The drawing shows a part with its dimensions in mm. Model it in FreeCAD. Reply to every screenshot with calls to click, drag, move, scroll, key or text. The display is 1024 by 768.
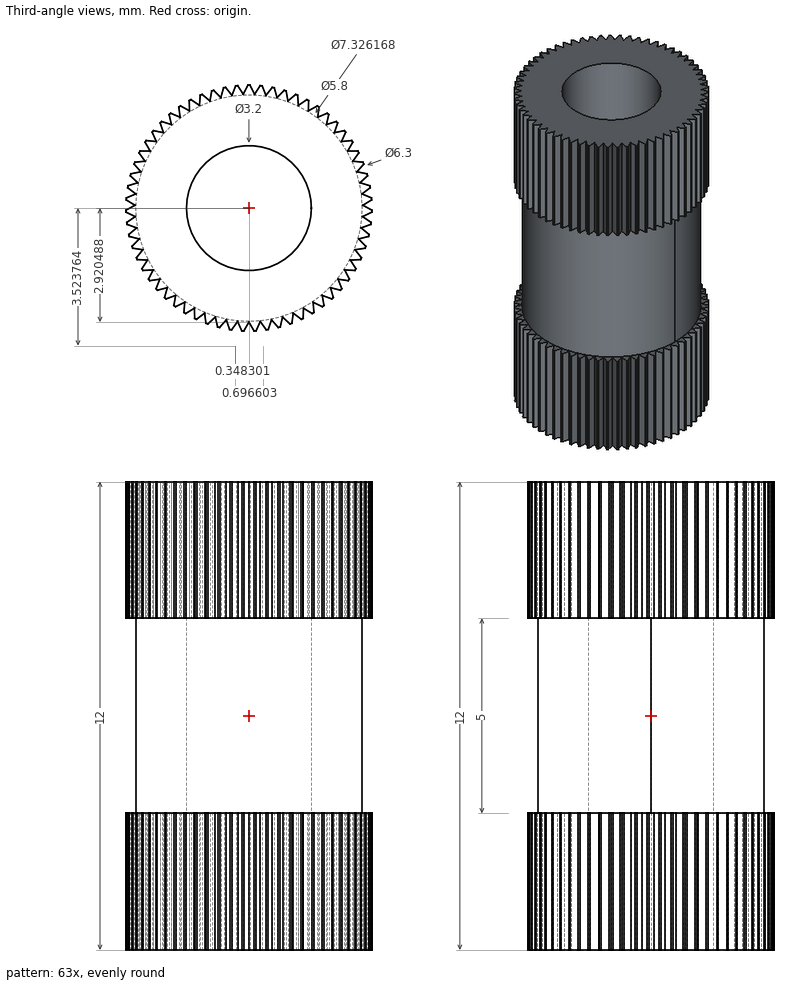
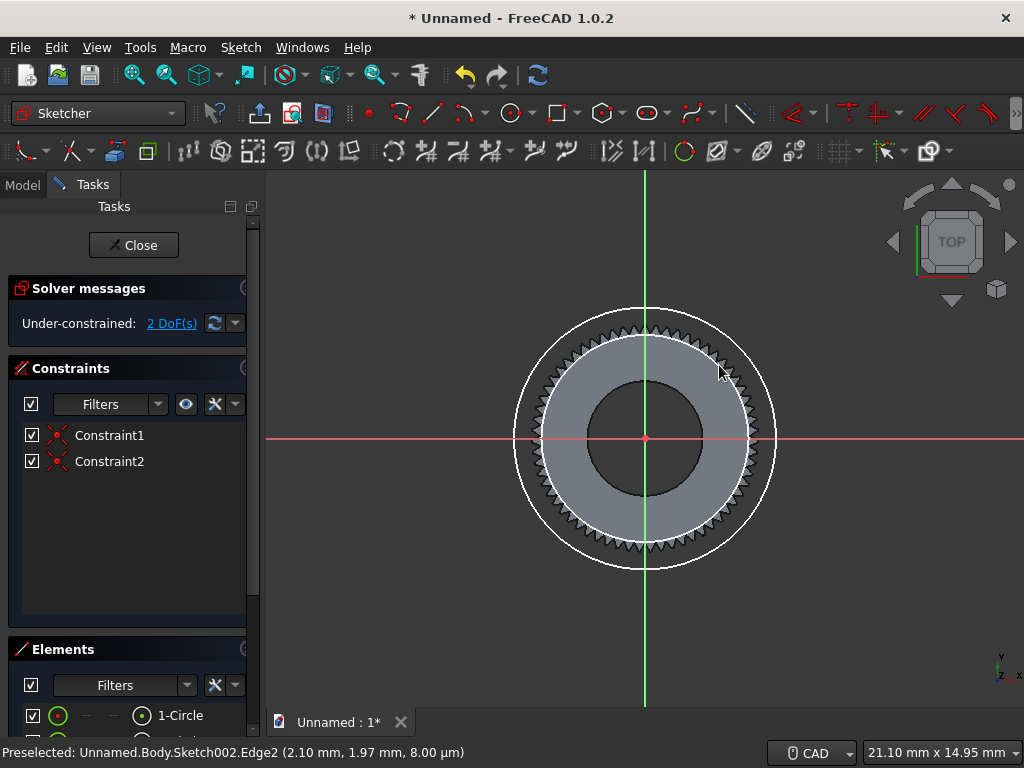
click(792, 114)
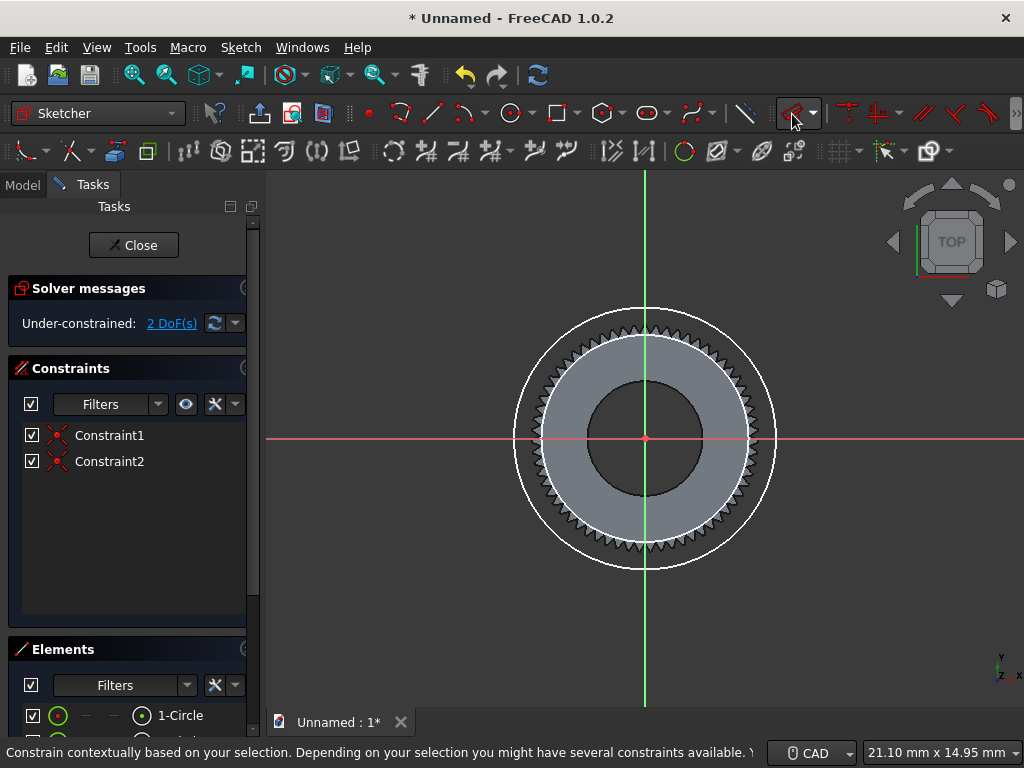
click(737, 345)
click(759, 322)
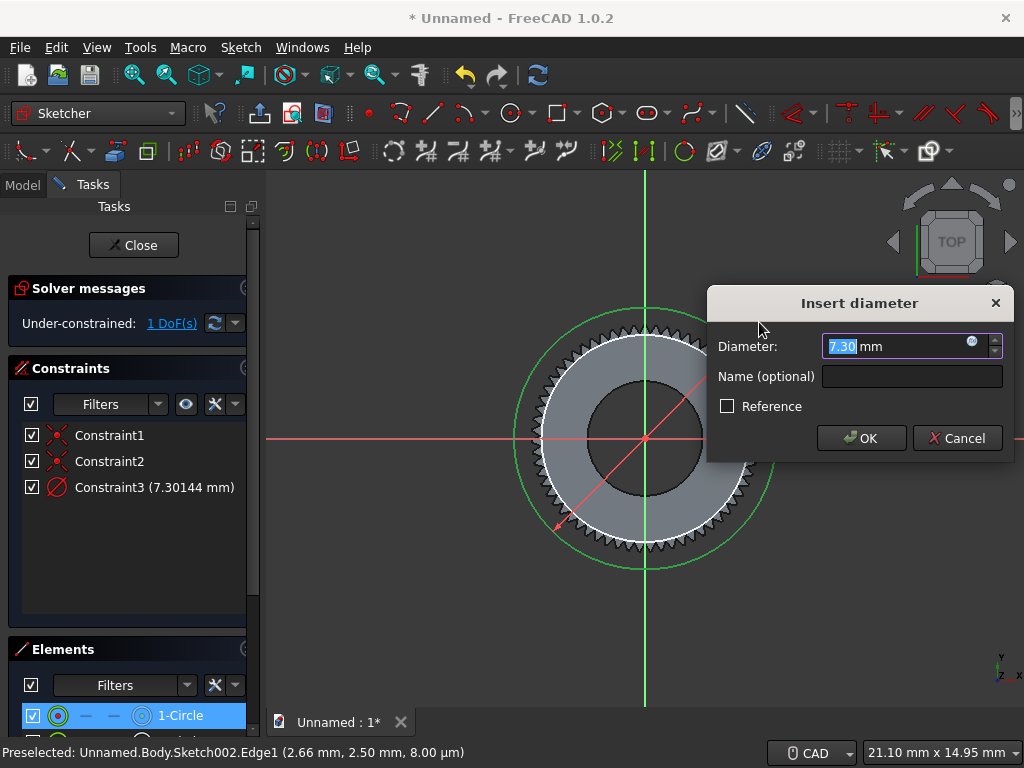
text(7.326168)
key(Return)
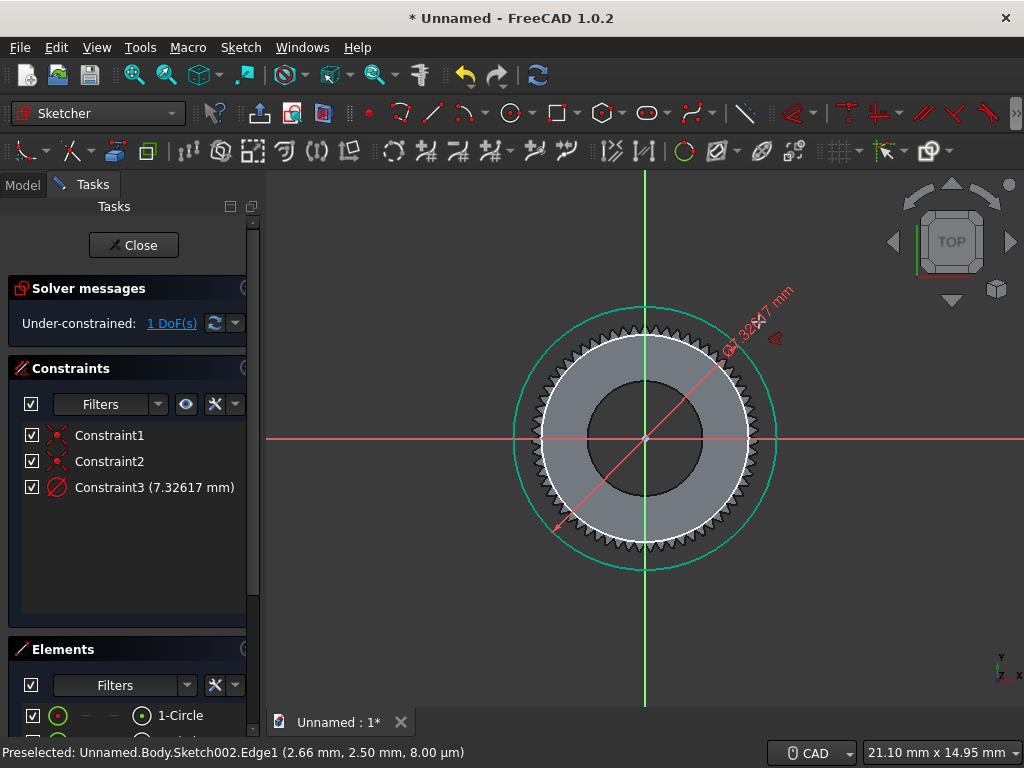
click(718, 365)
click(797, 393)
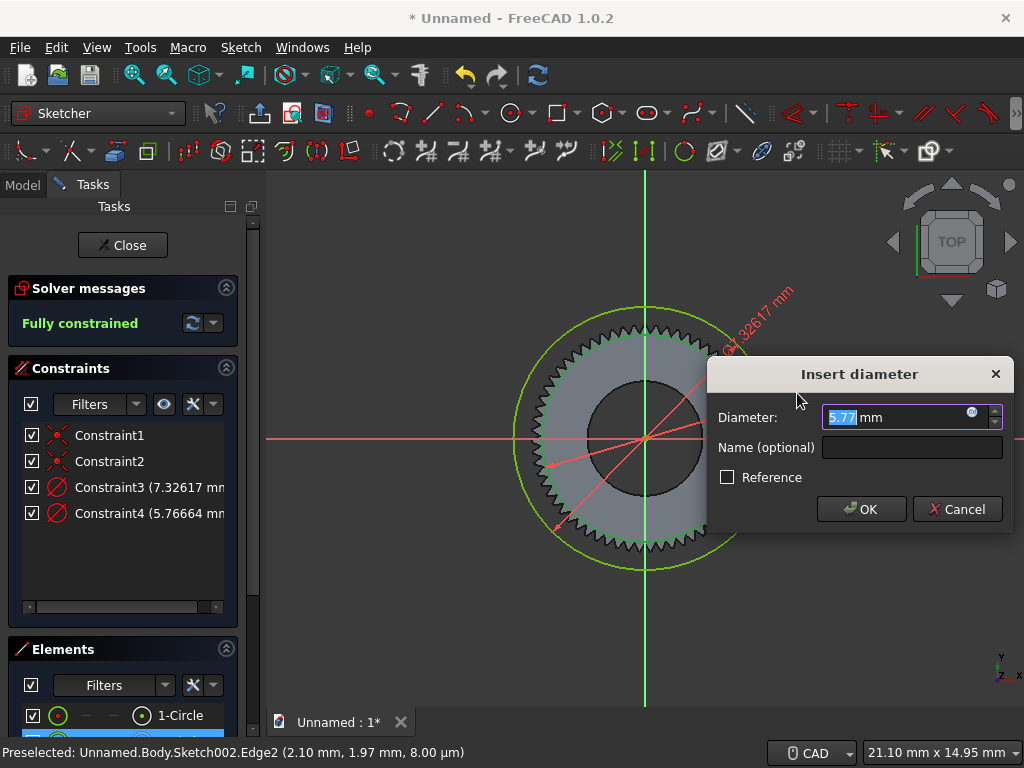
text(5.8)
key(Return)
key(Escape)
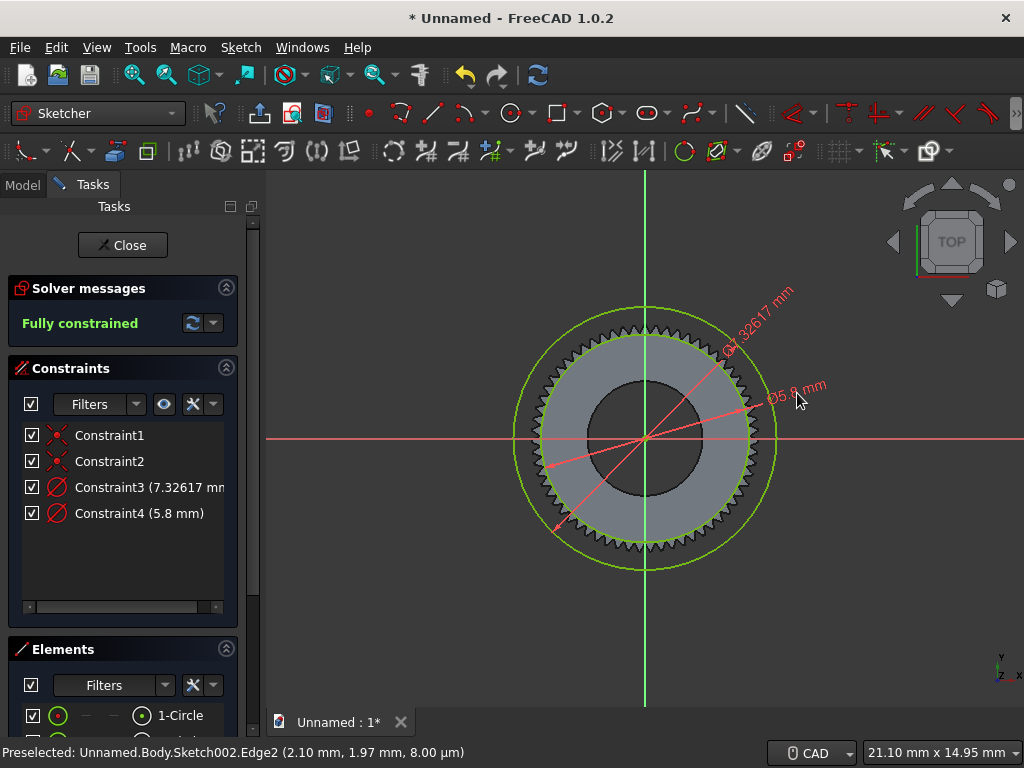
click(123, 245)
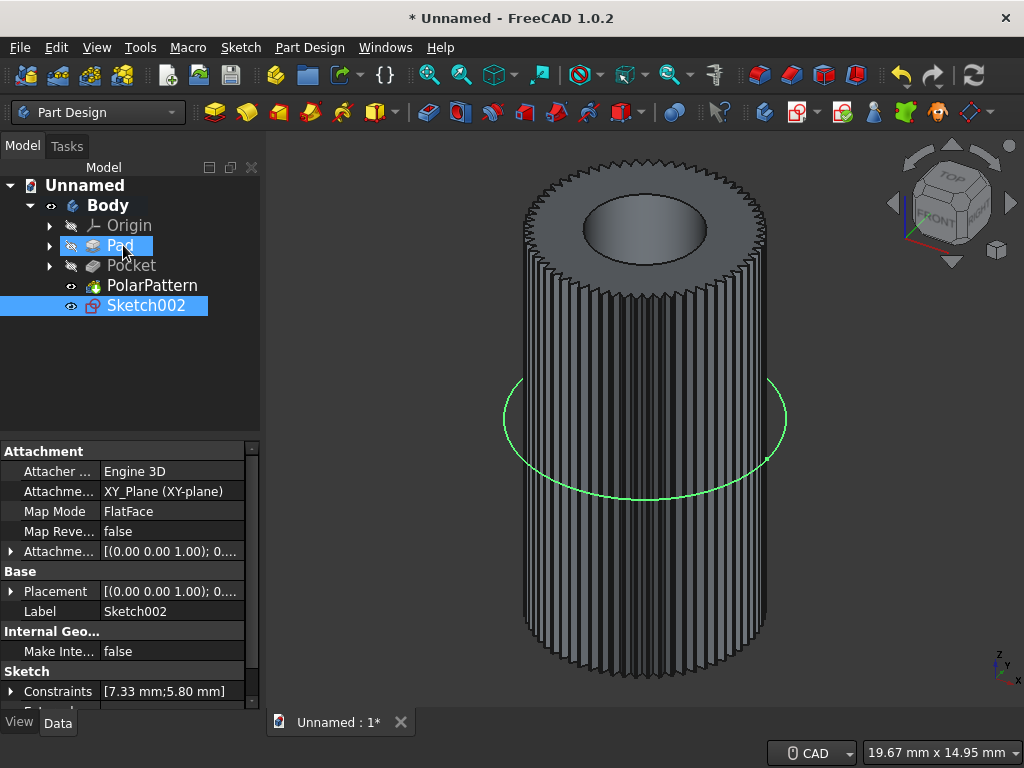
click(430, 112)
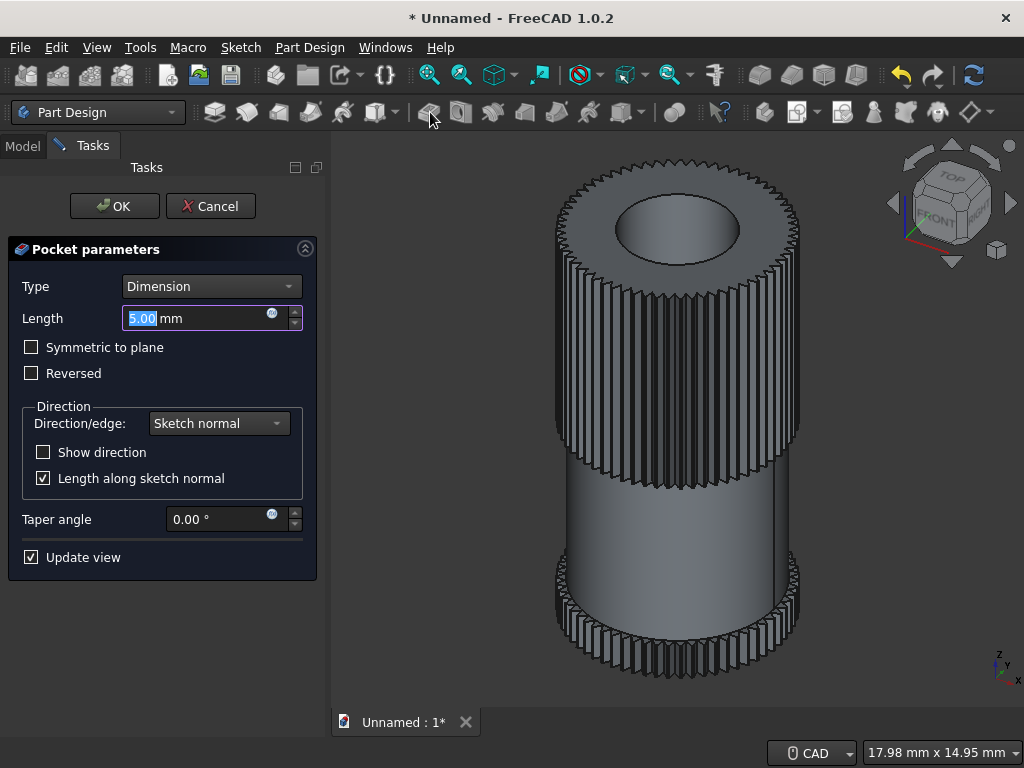
text(5)
key(Tab)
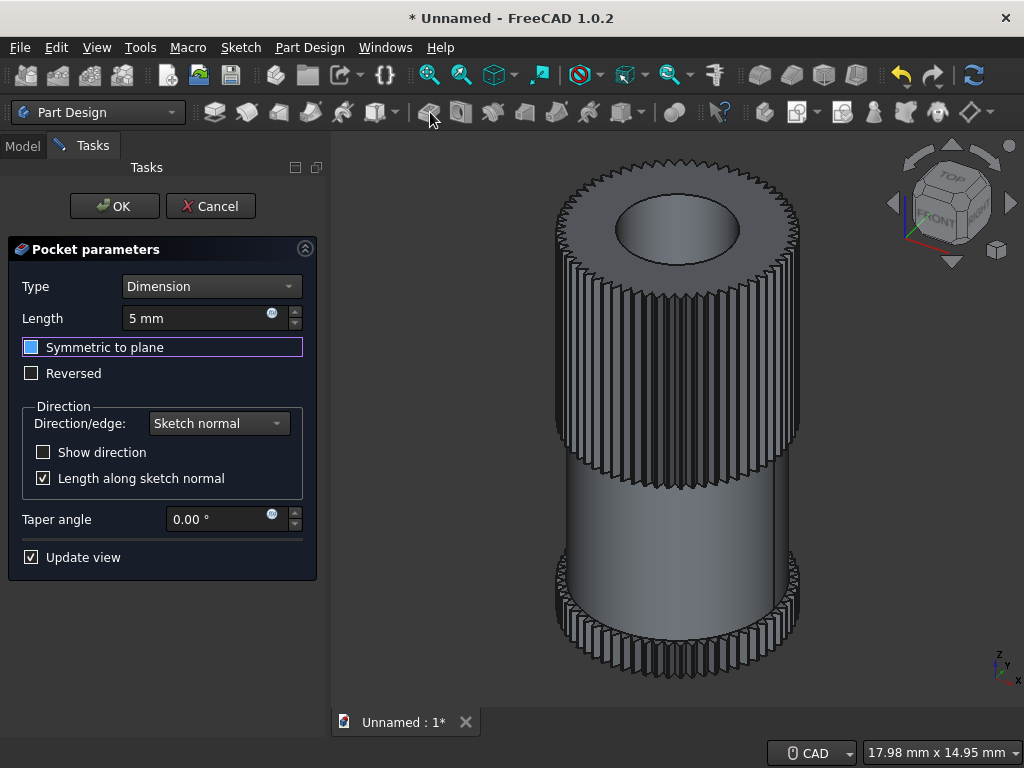
click(30, 347)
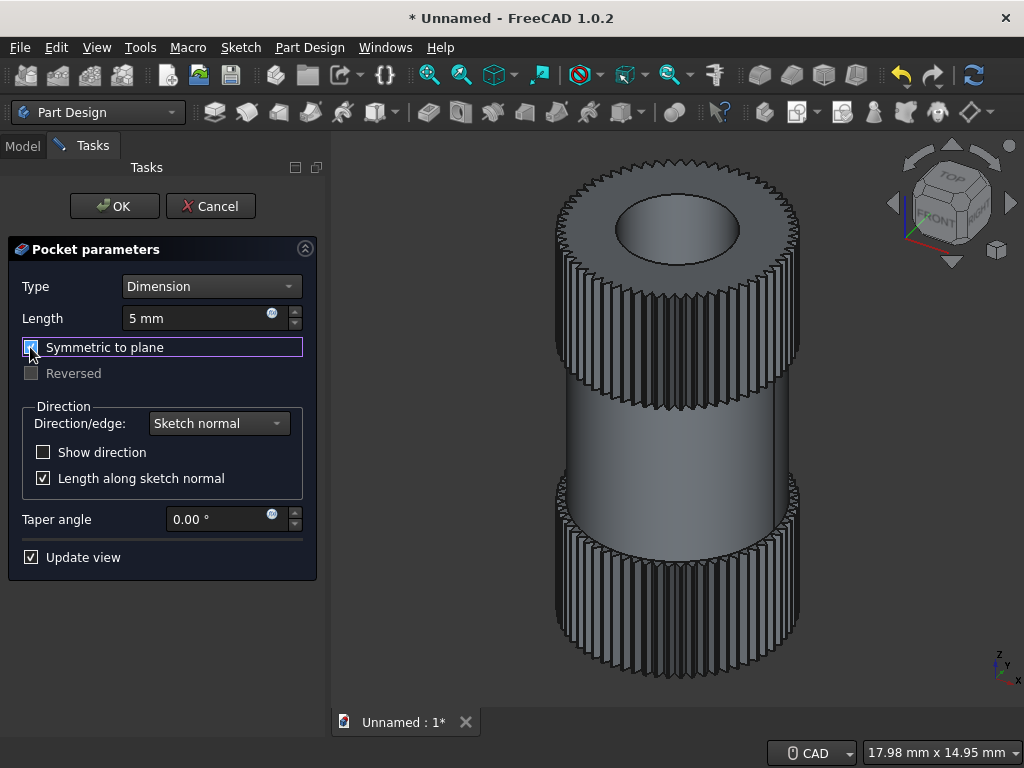
click(115, 206)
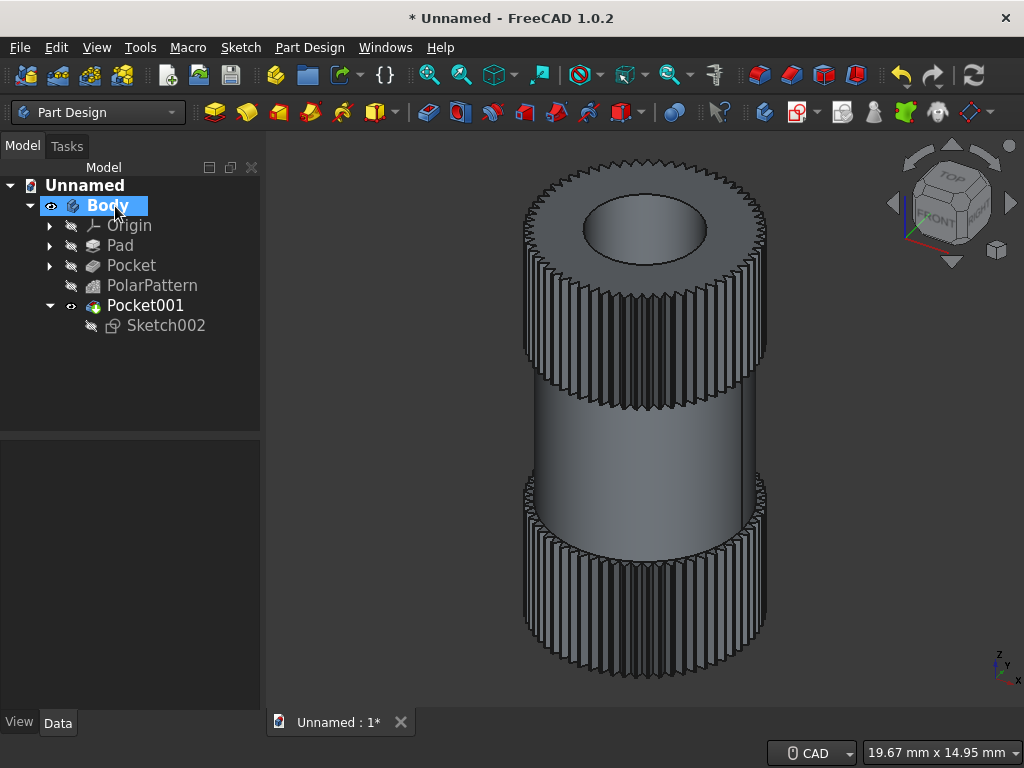
key(0)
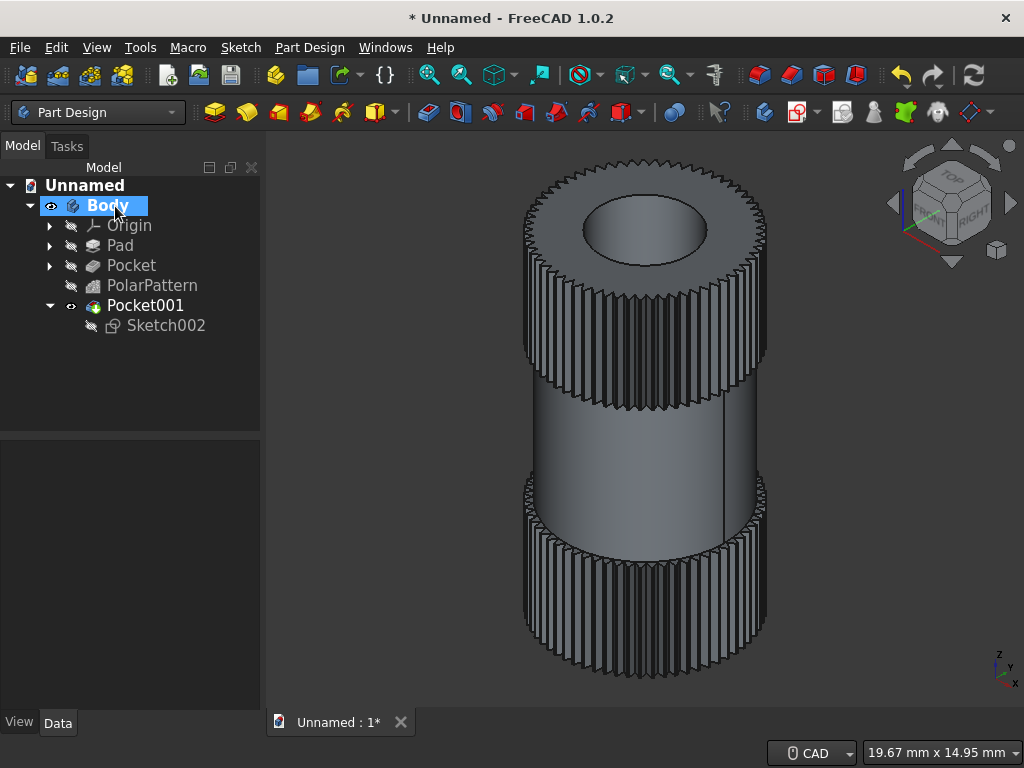
click(430, 76)